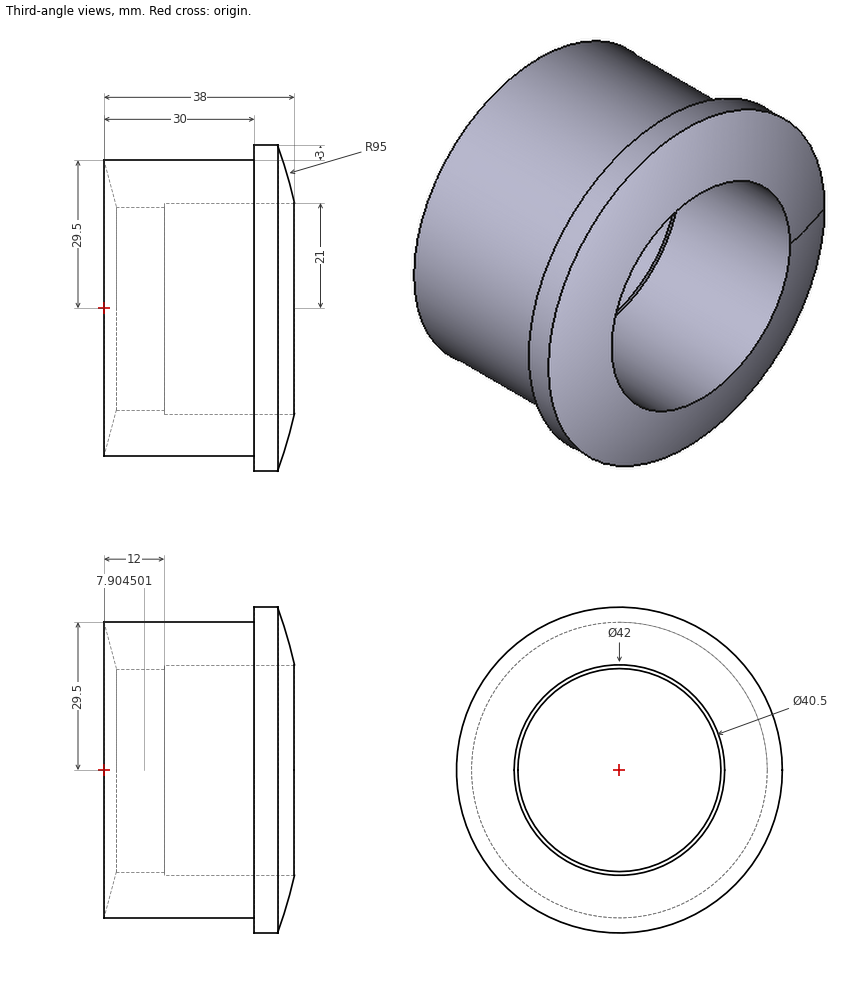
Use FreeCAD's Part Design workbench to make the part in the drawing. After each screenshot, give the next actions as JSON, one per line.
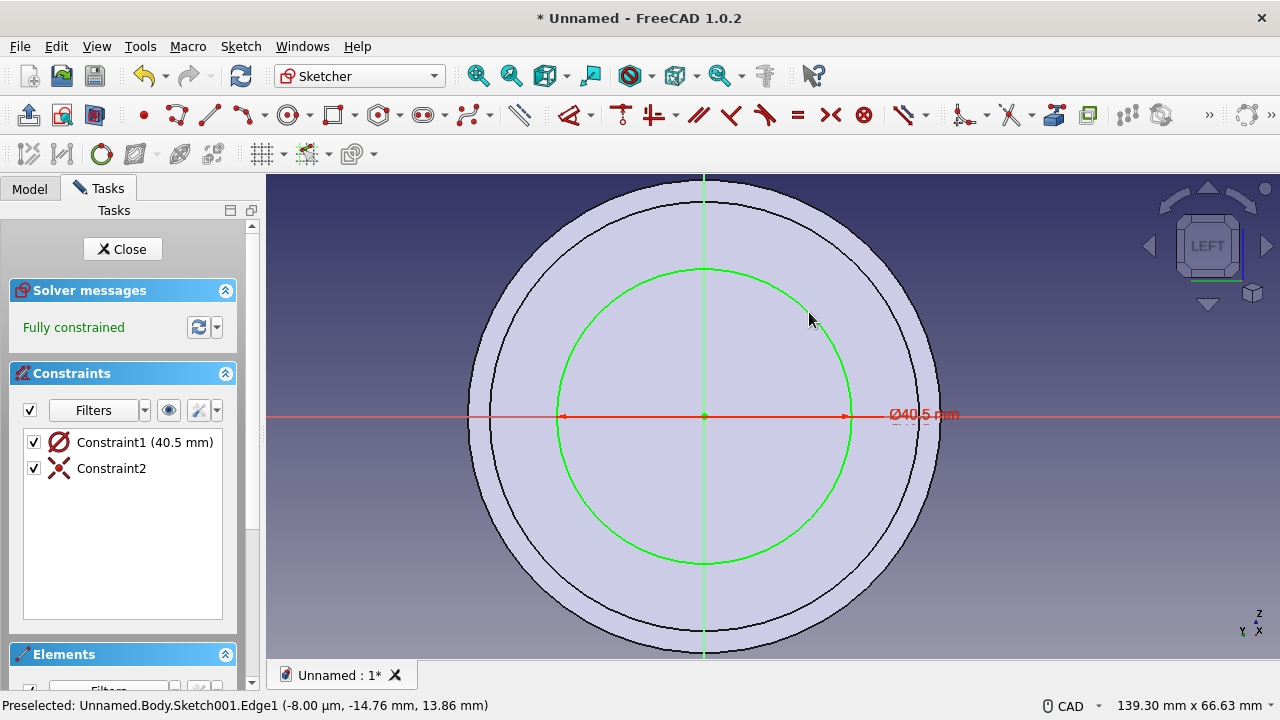
{"action": "left_click", "coordinate": [123, 249]}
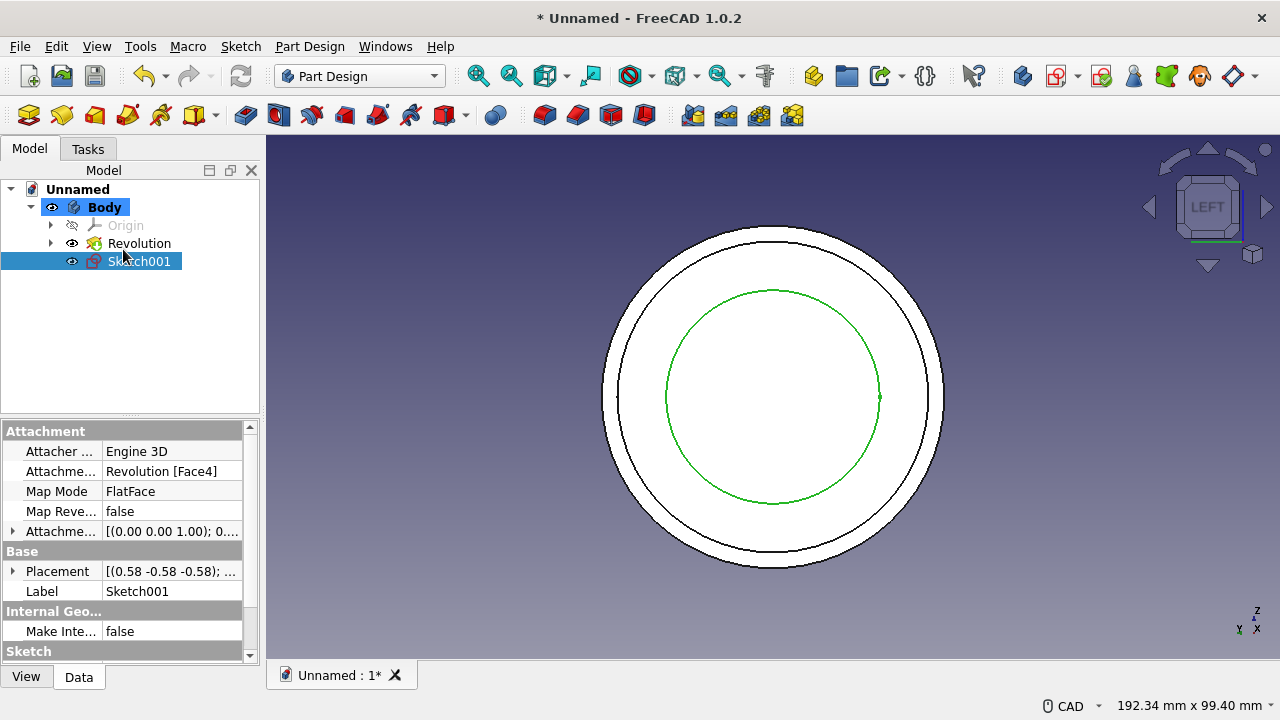
{"action": "left_click", "coordinate": [246, 116]}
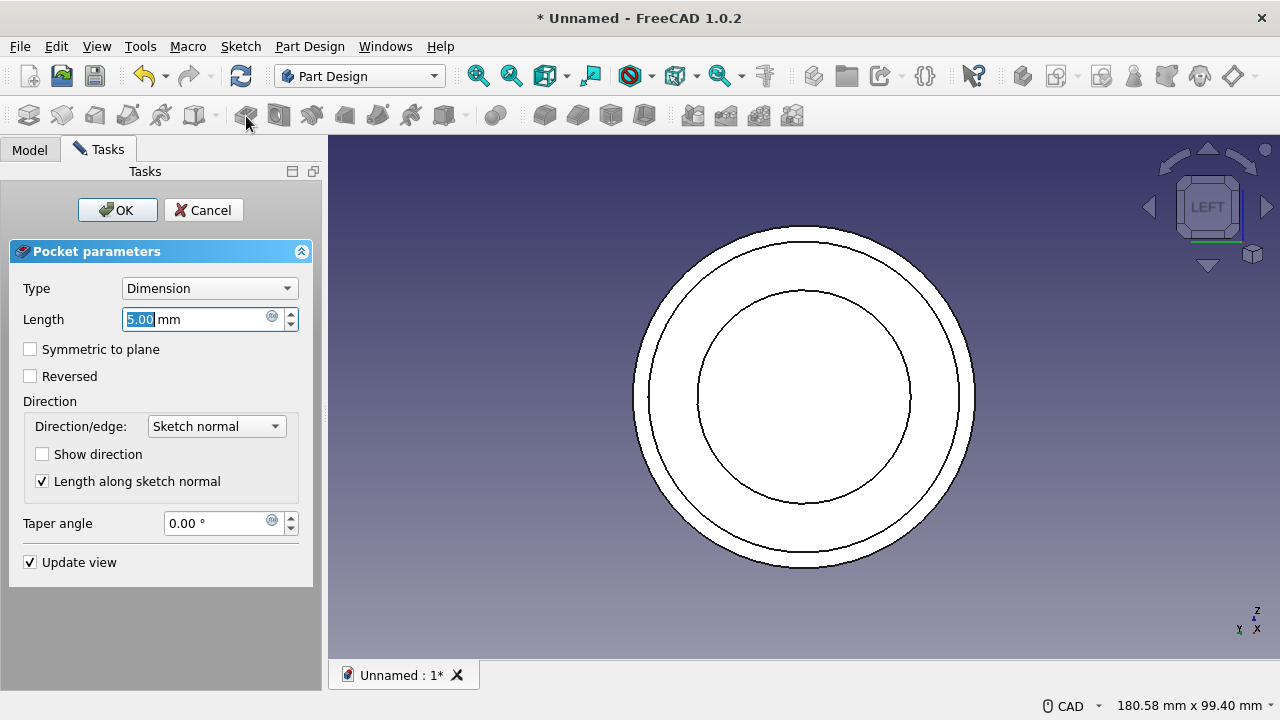
{"action": "type", "text": "12"}
{"action": "key", "text": "Tab"}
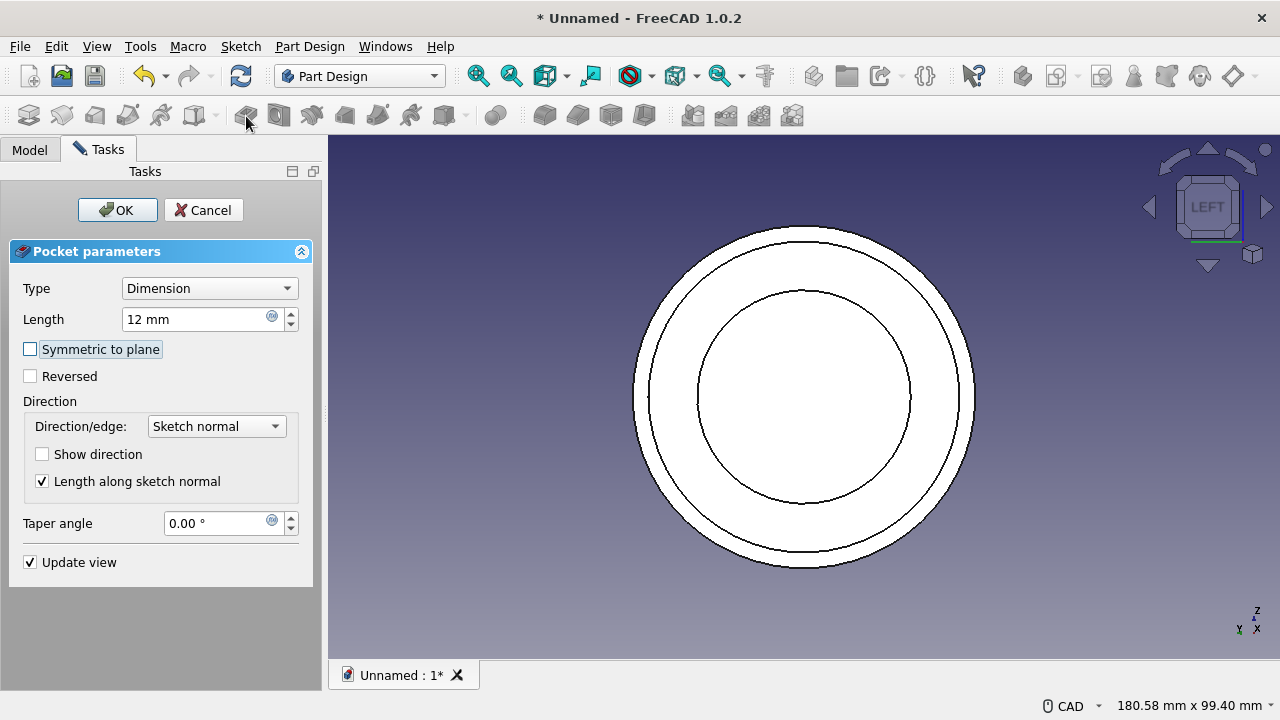
{"action": "left_click", "coordinate": [118, 210]}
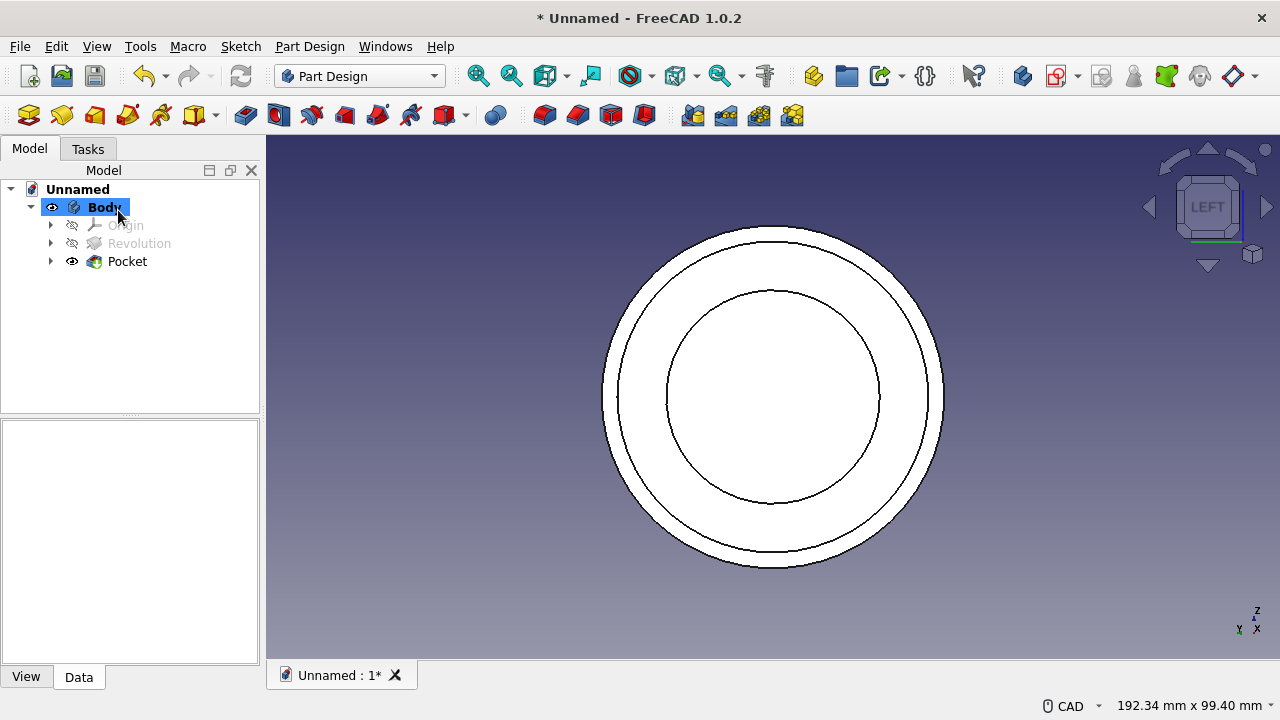
{"action": "left_click", "coordinate": [1056, 76]}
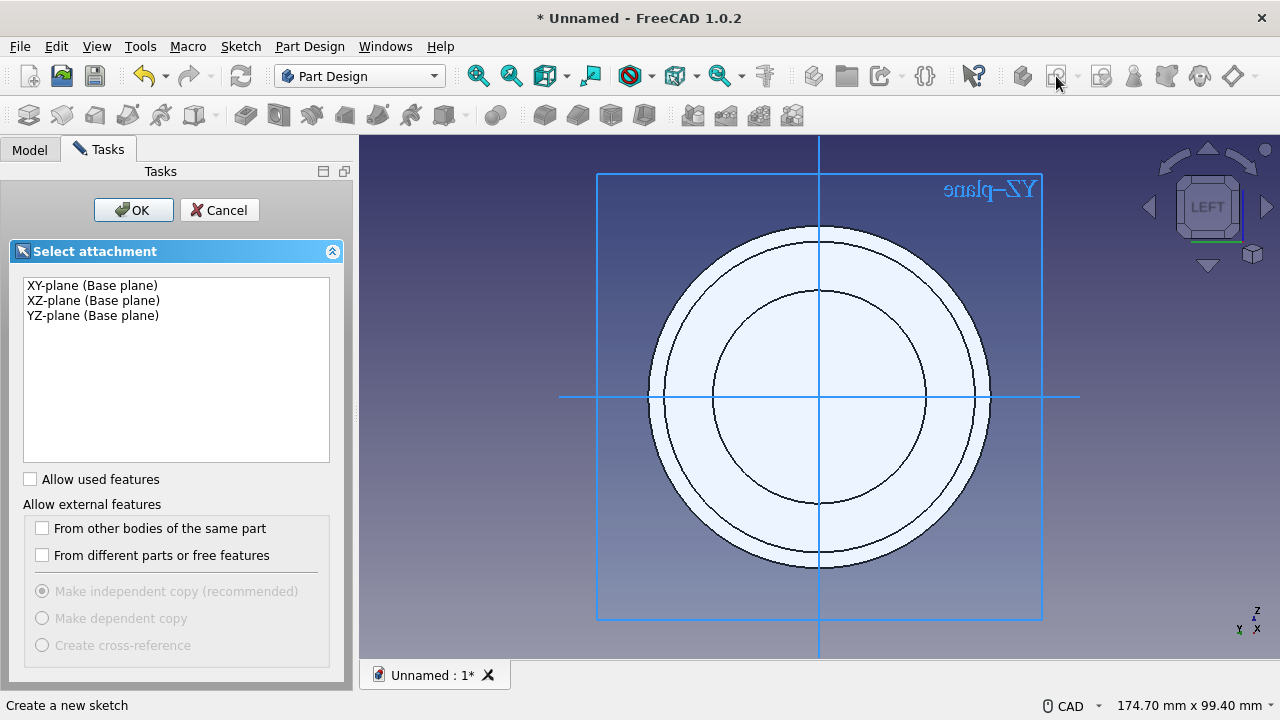
{"action": "left_click", "coordinate": [84, 300]}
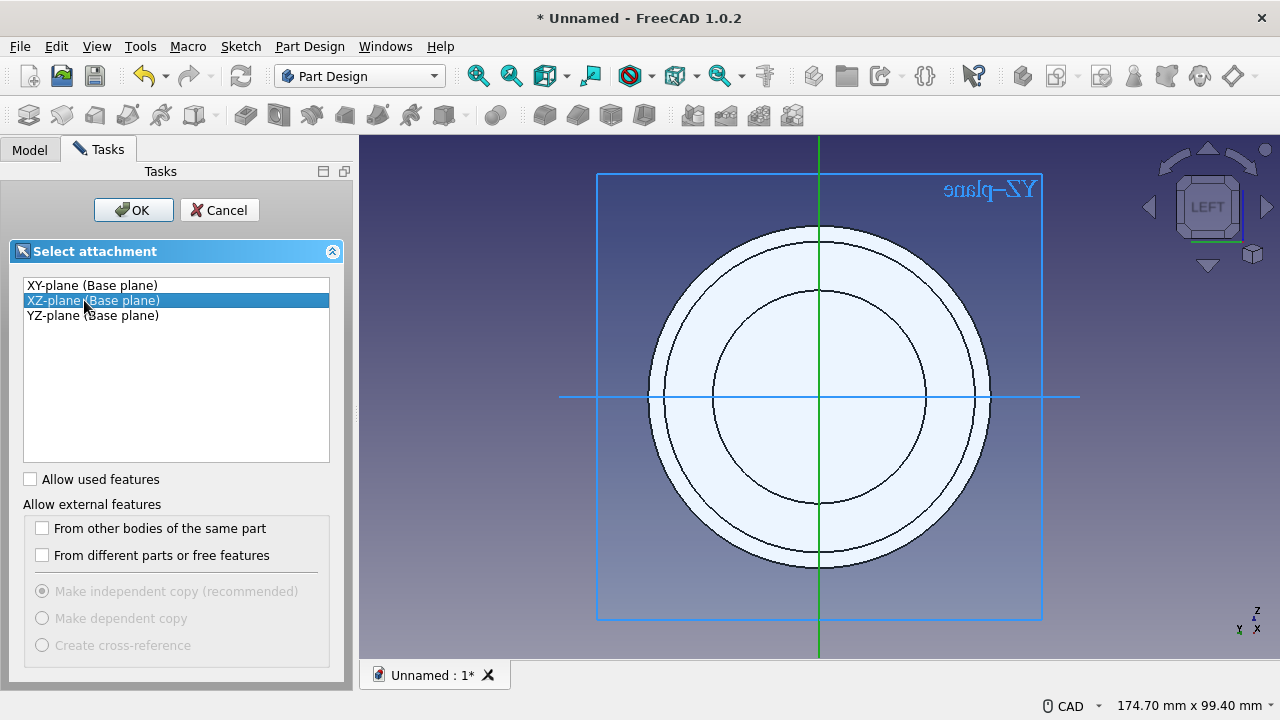
{"action": "left_click", "coordinate": [134, 210]}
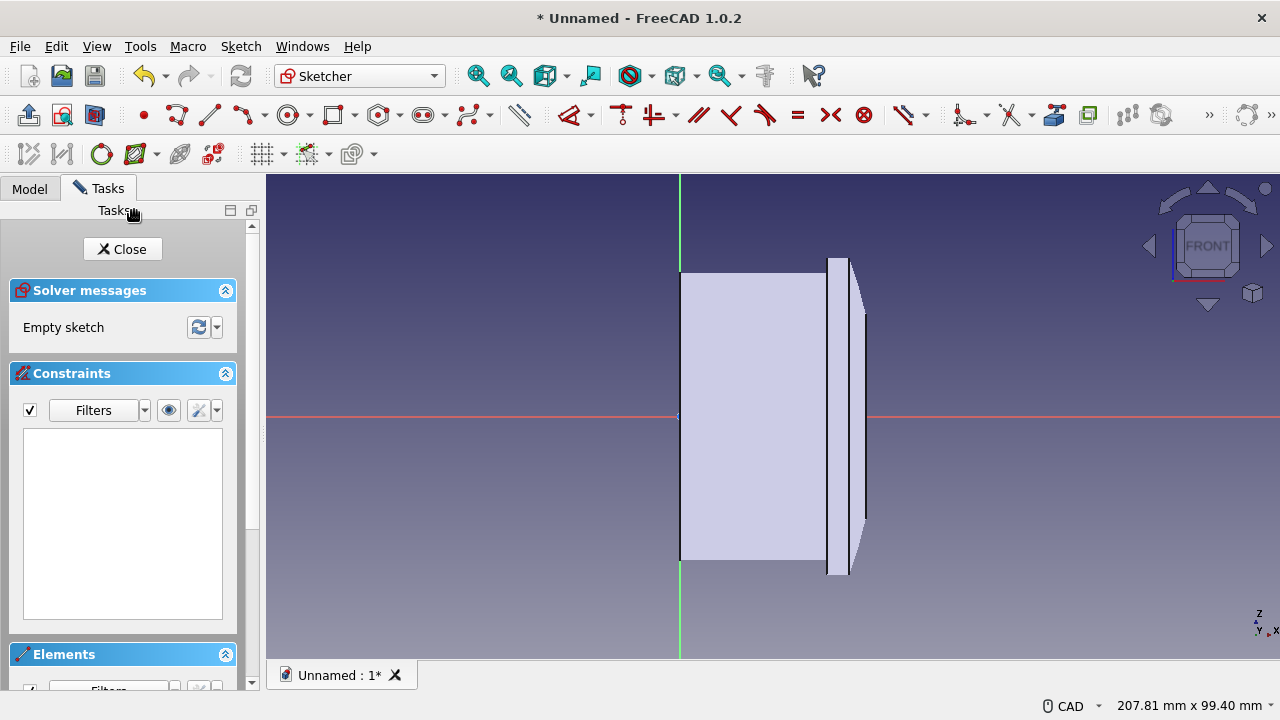
{"action": "left_click", "coordinate": [95, 116]}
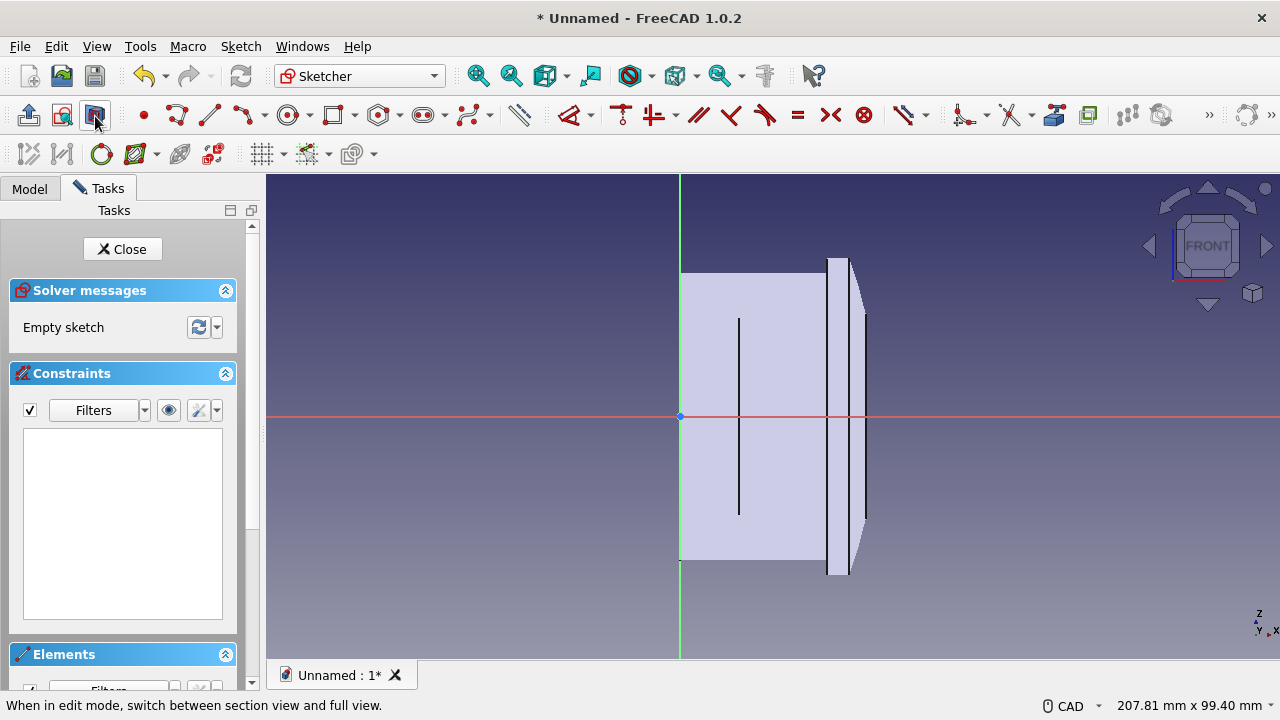
{"action": "scroll", "coordinate": [696, 286], "scroll_direction": "up", "scroll_amount": 4}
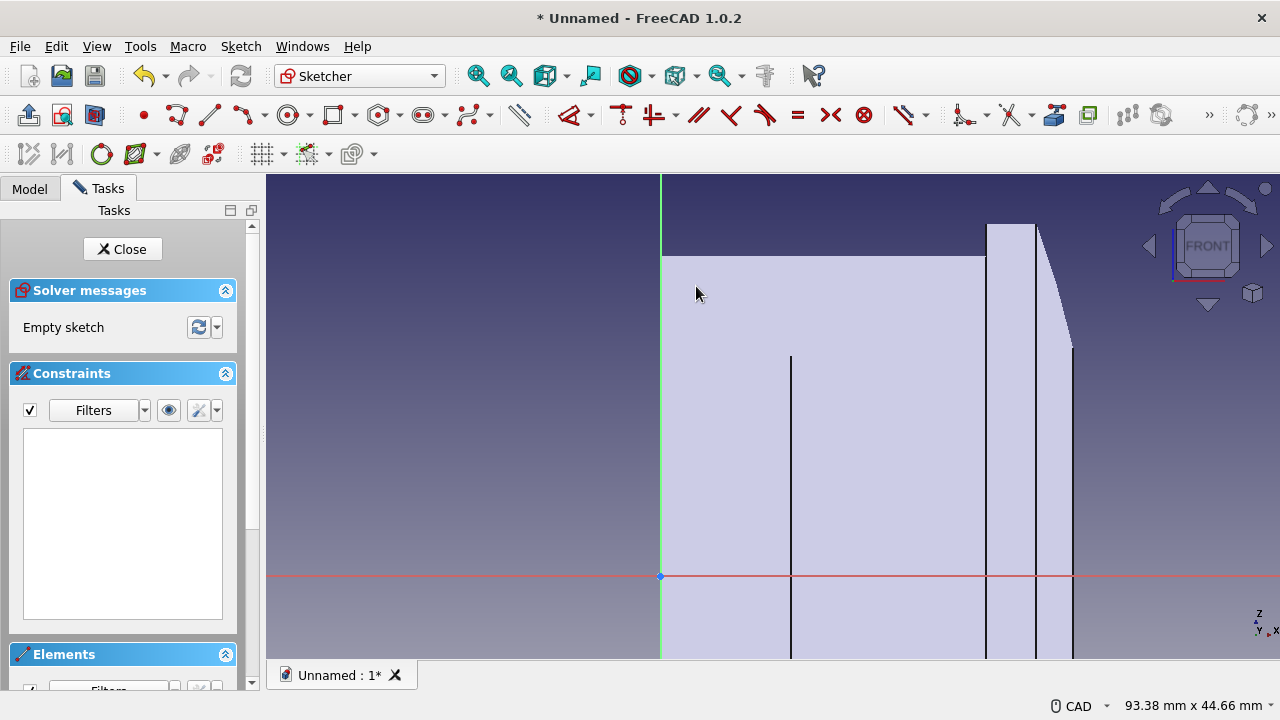
{"action": "left_click", "coordinate": [177, 116]}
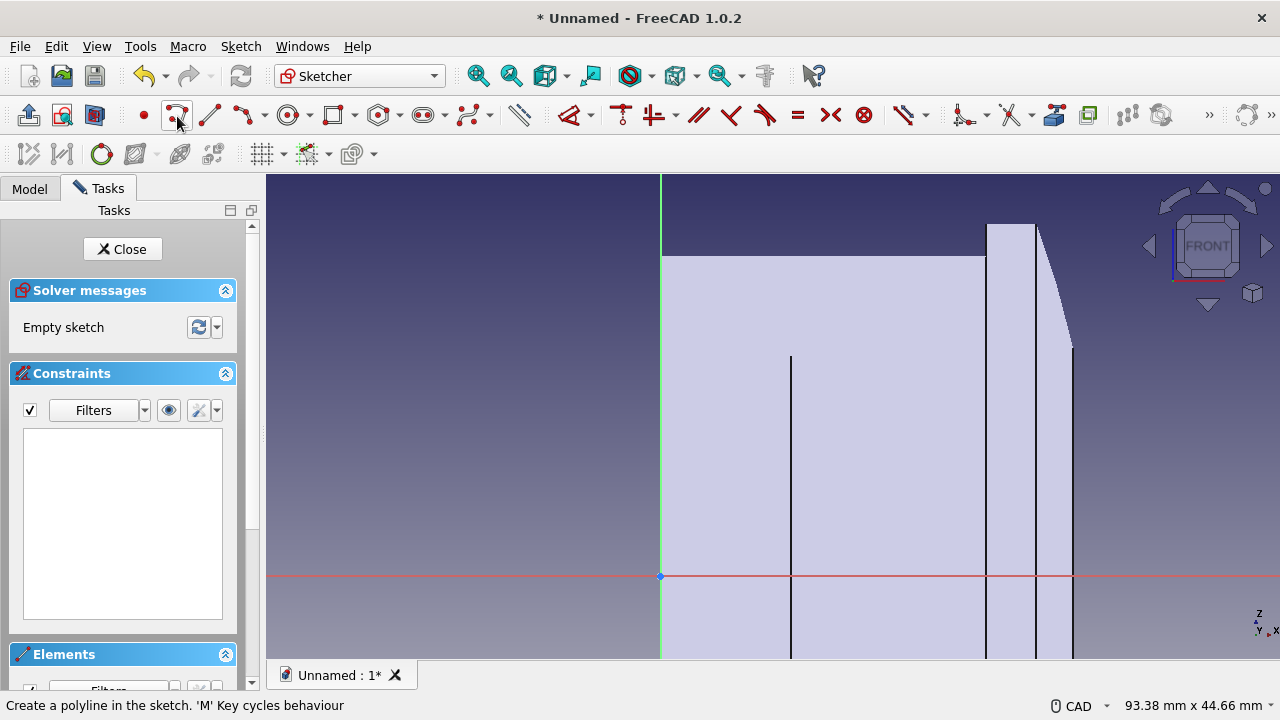
{"action": "left_click", "coordinate": [661, 576]}
{"action": "left_click", "coordinate": [670, 256]}
{"action": "left_click", "coordinate": [746, 567]}
{"action": "left_click", "coordinate": [661, 576]}
{"action": "key", "text": "Escape"}
{"action": "key", "text": "Escape"}